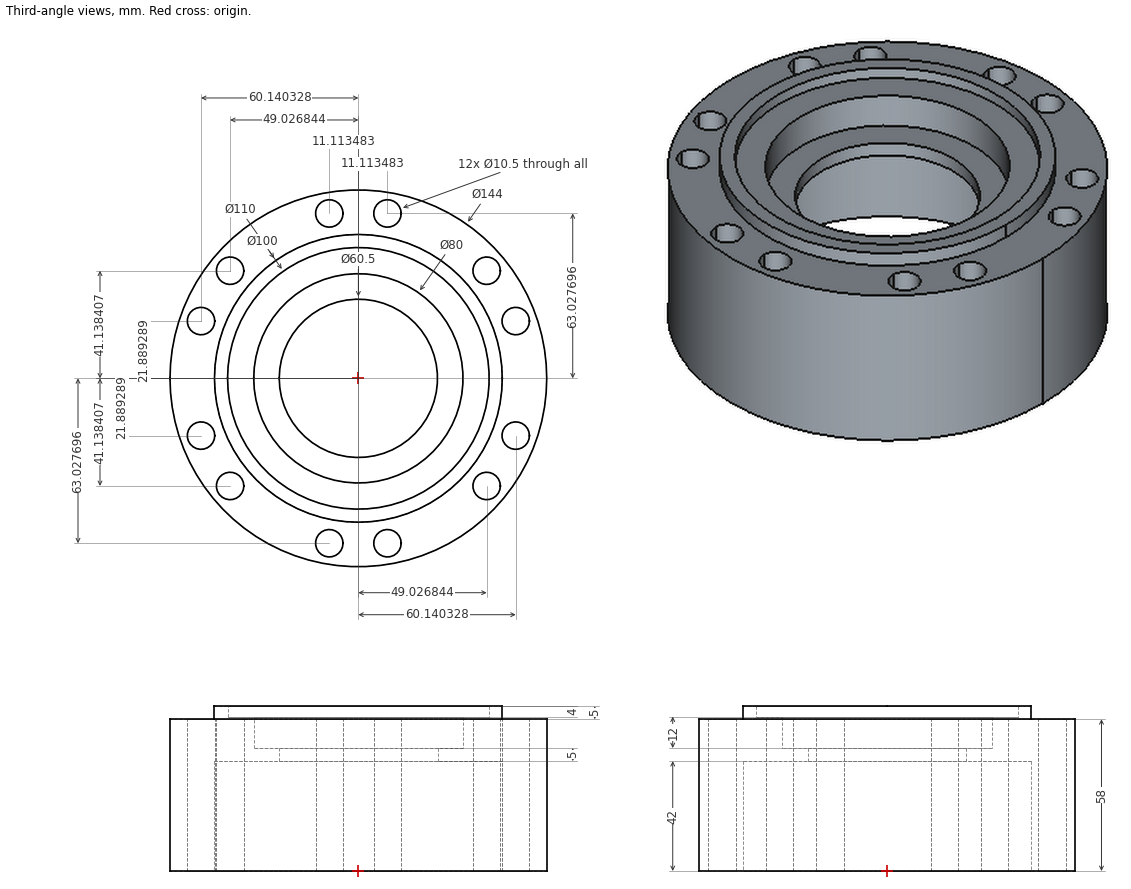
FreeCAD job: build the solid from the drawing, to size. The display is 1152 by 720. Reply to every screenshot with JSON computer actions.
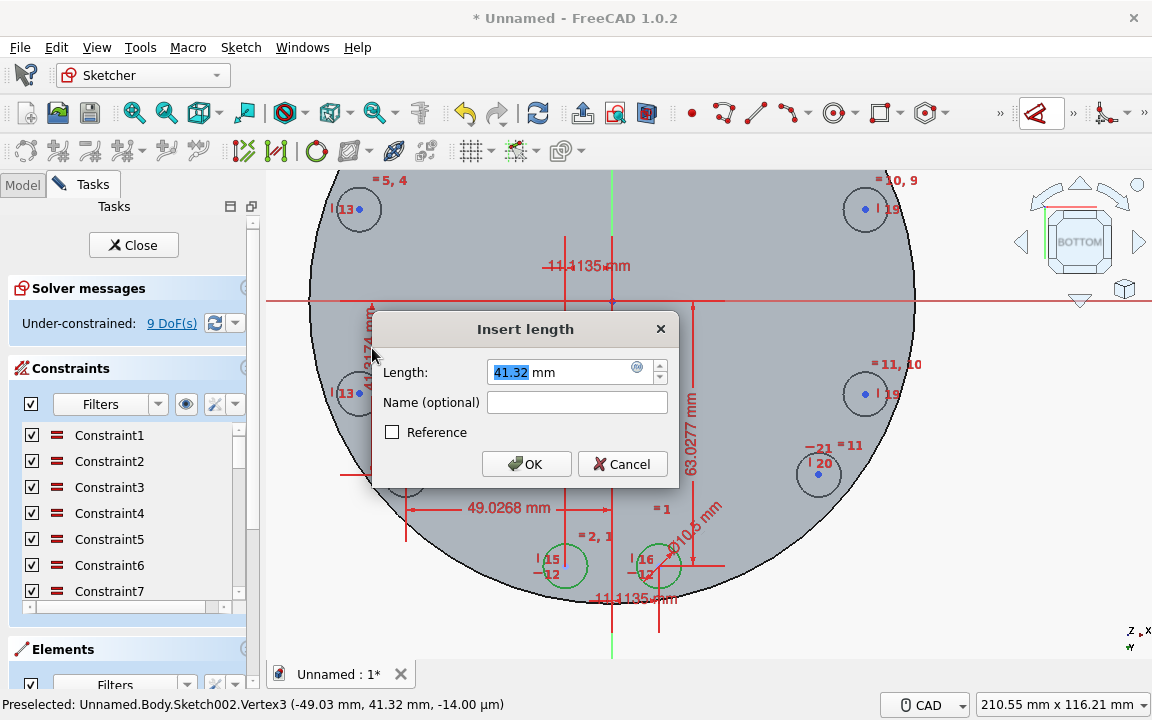
{"action": "type", "text": "41.138407"}
{"action": "key", "text": "Return"}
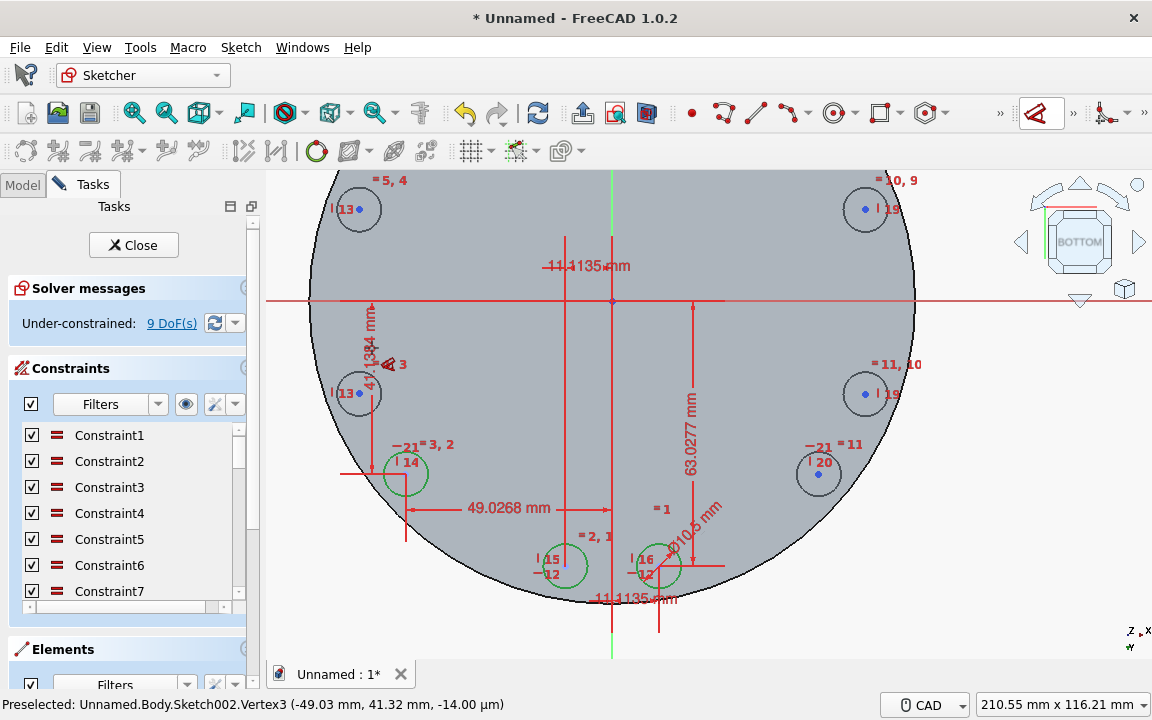
{"action": "left_click", "coordinate": [359, 394]}
{"action": "left_click", "coordinate": [486, 428]}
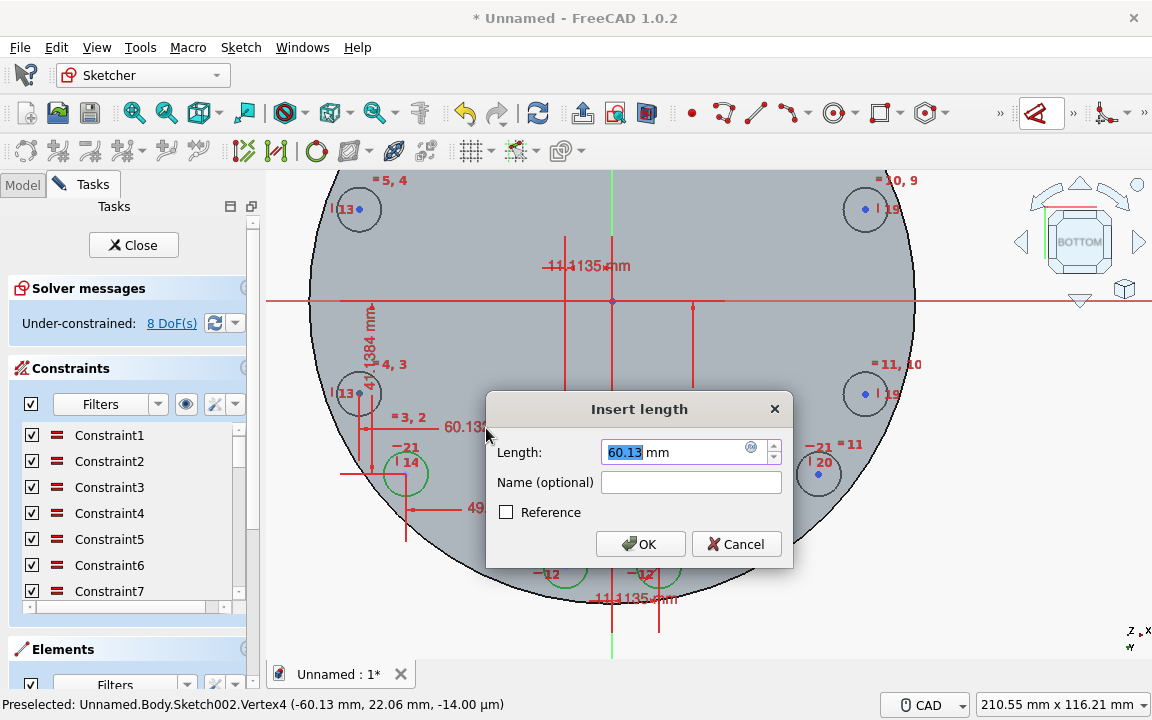
{"action": "type", "text": "60.140328"}
{"action": "key", "text": "Return"}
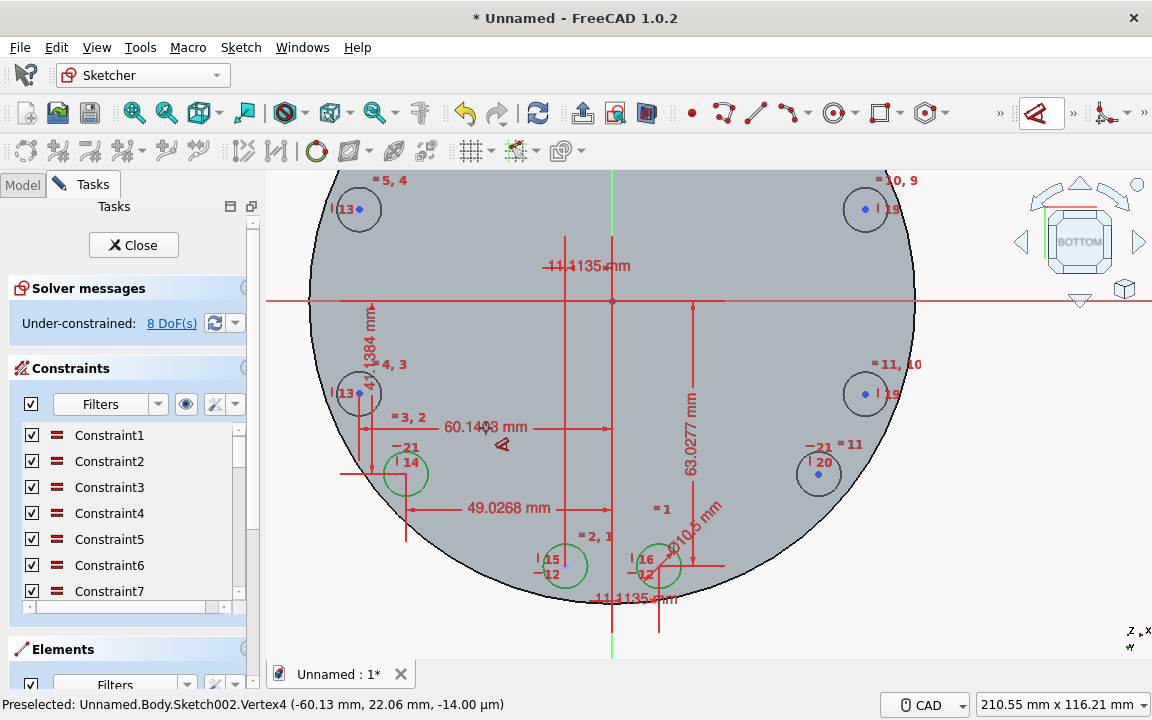
{"action": "left_click", "coordinate": [359, 394]}
{"action": "left_click", "coordinate": [325, 326]}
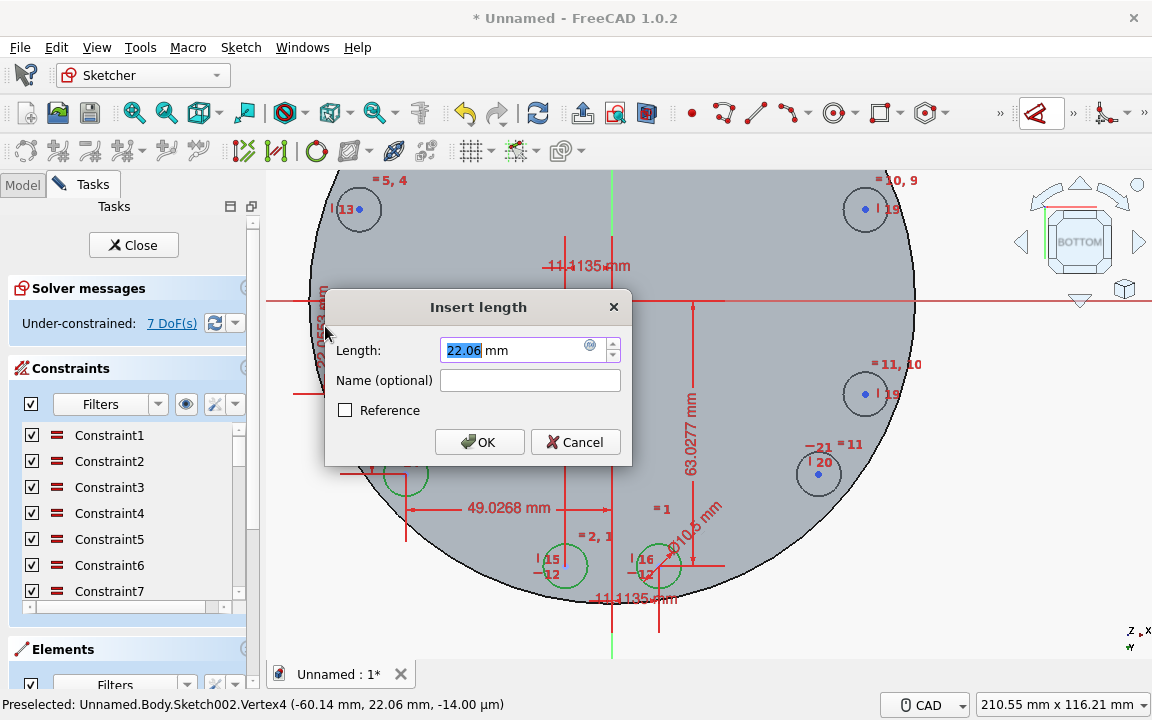
{"action": "type", "text": "21.889289"}
{"action": "key", "text": "Return"}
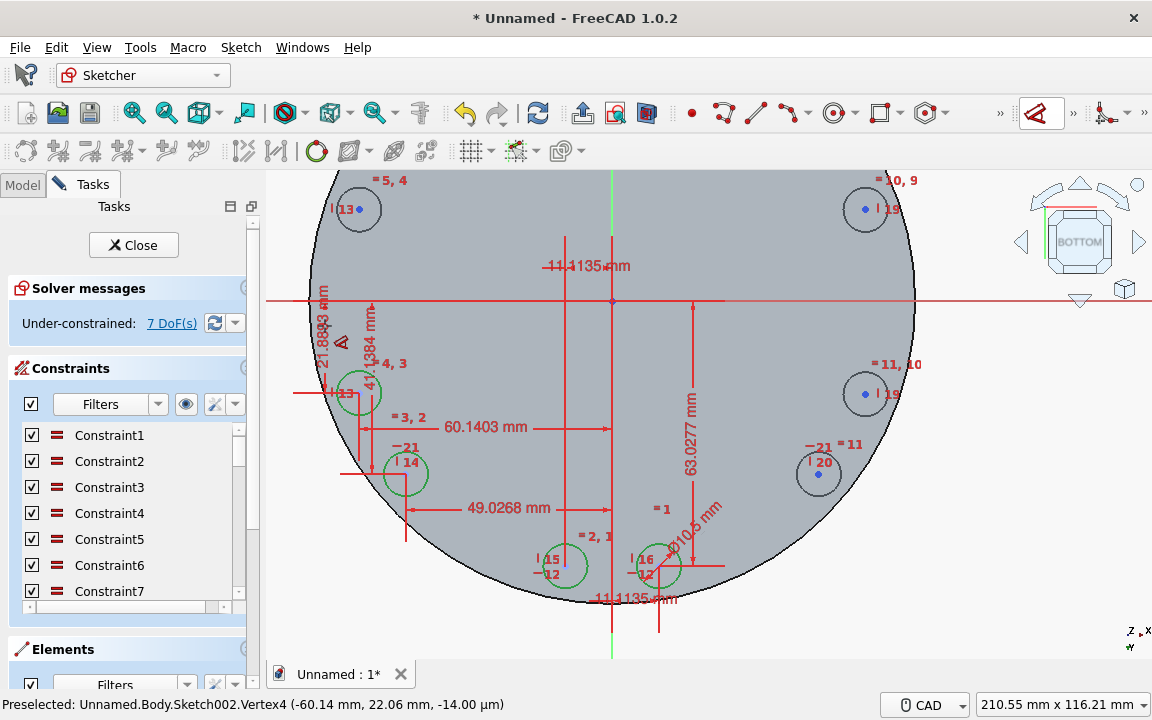
{"action": "left_click", "coordinate": [359, 210]}
{"action": "left_click", "coordinate": [325, 255]}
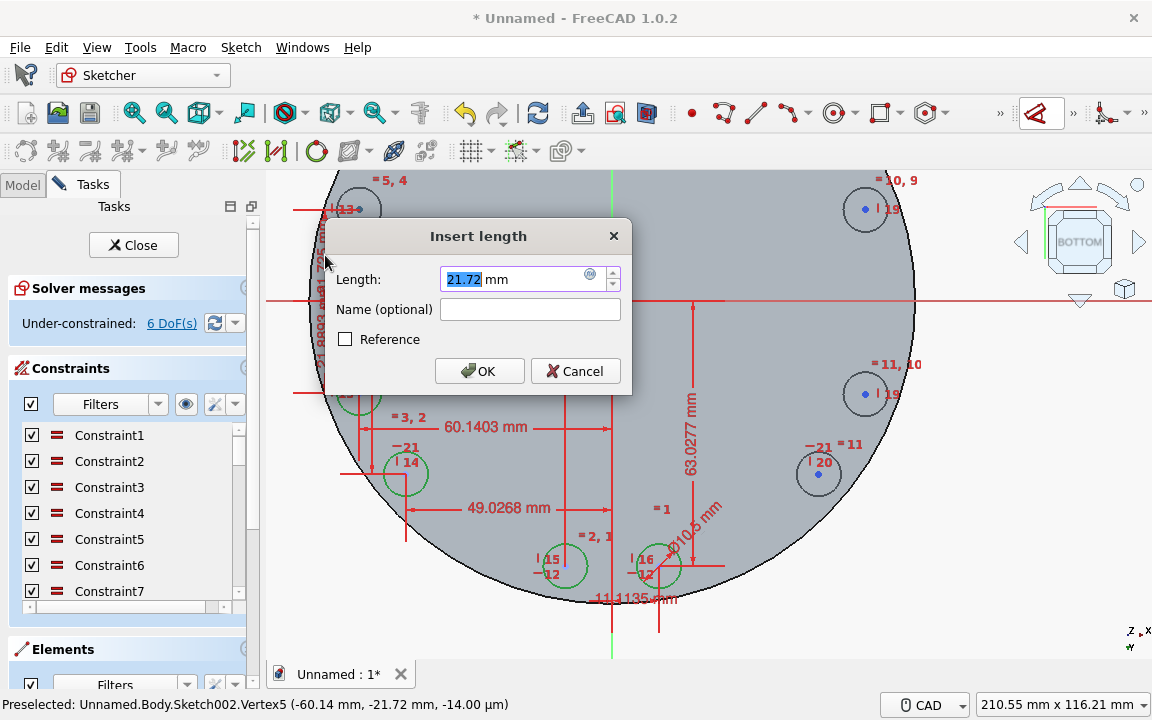
{"action": "type", "text": "21.889289"}
{"action": "key", "text": "Return"}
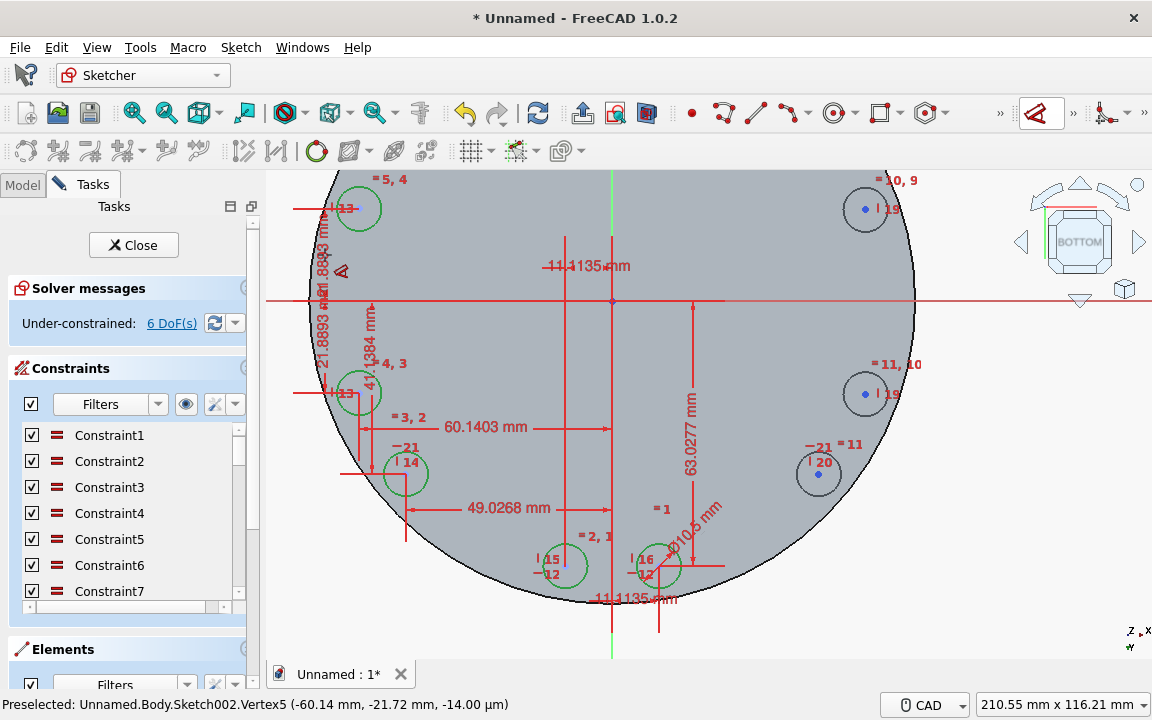
{"action": "scroll", "coordinate": [675, 553], "scroll_direction": "down", "scroll_amount": 3}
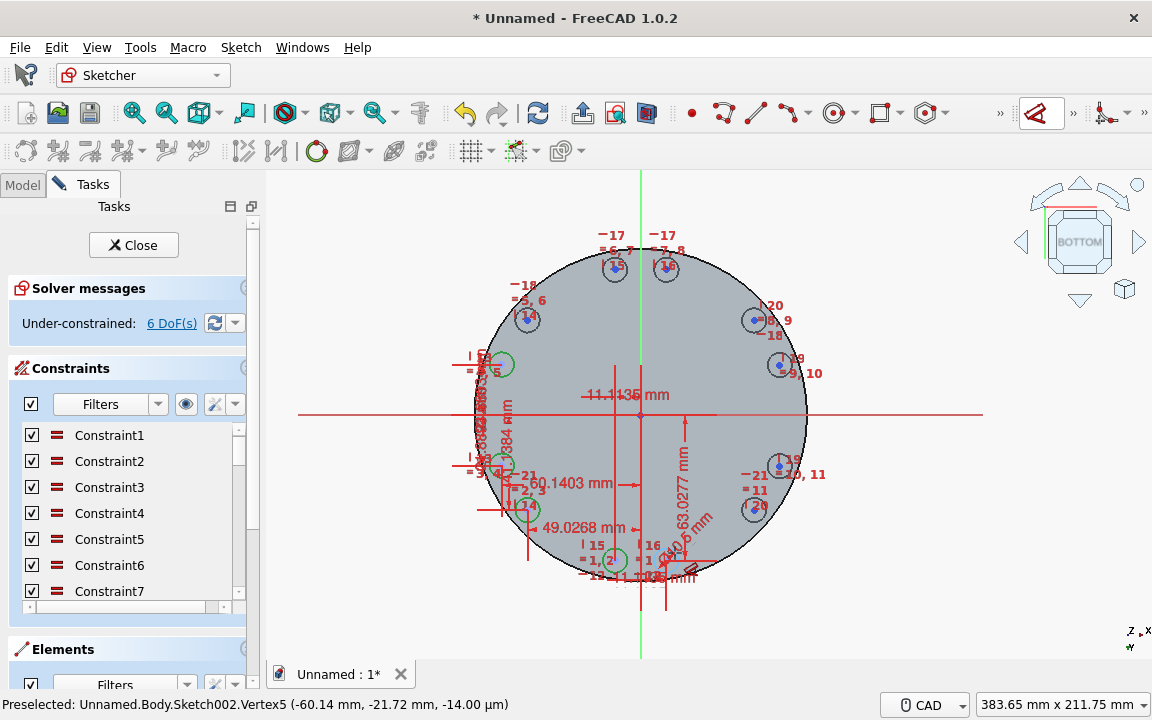
{"action": "left_click", "coordinate": [528, 320]}
{"action": "left_click", "coordinate": [494, 335]}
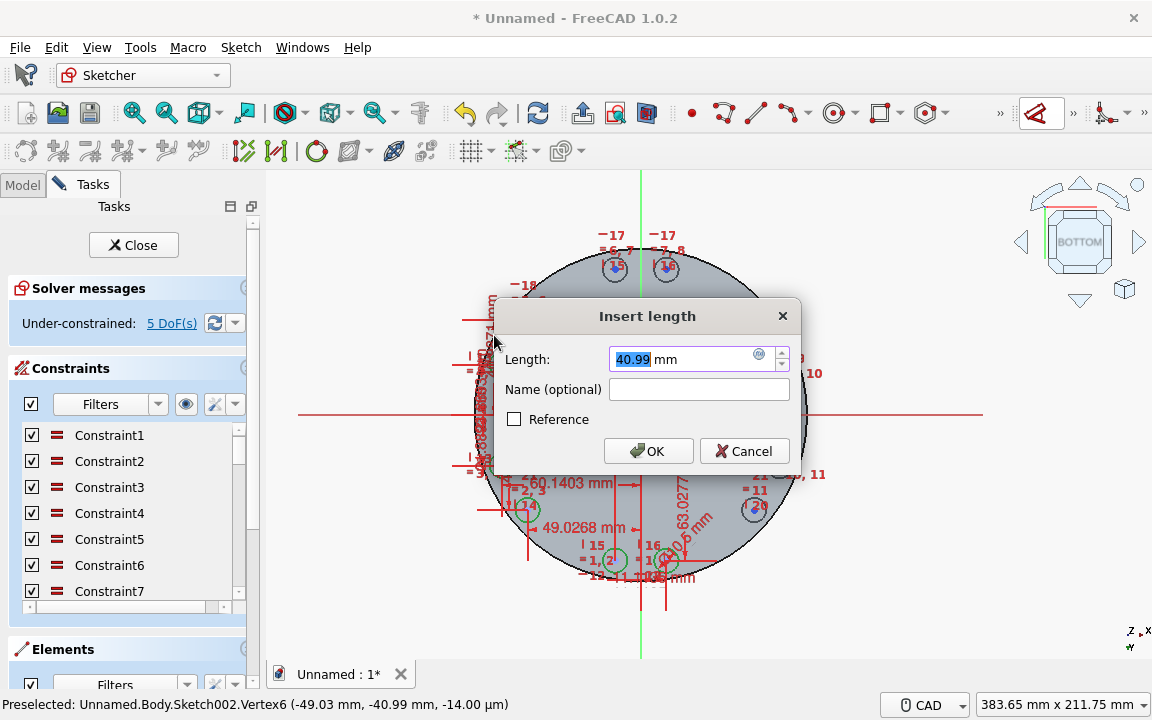
{"action": "type", "text": "41.138407"}
{"action": "key", "text": "Return"}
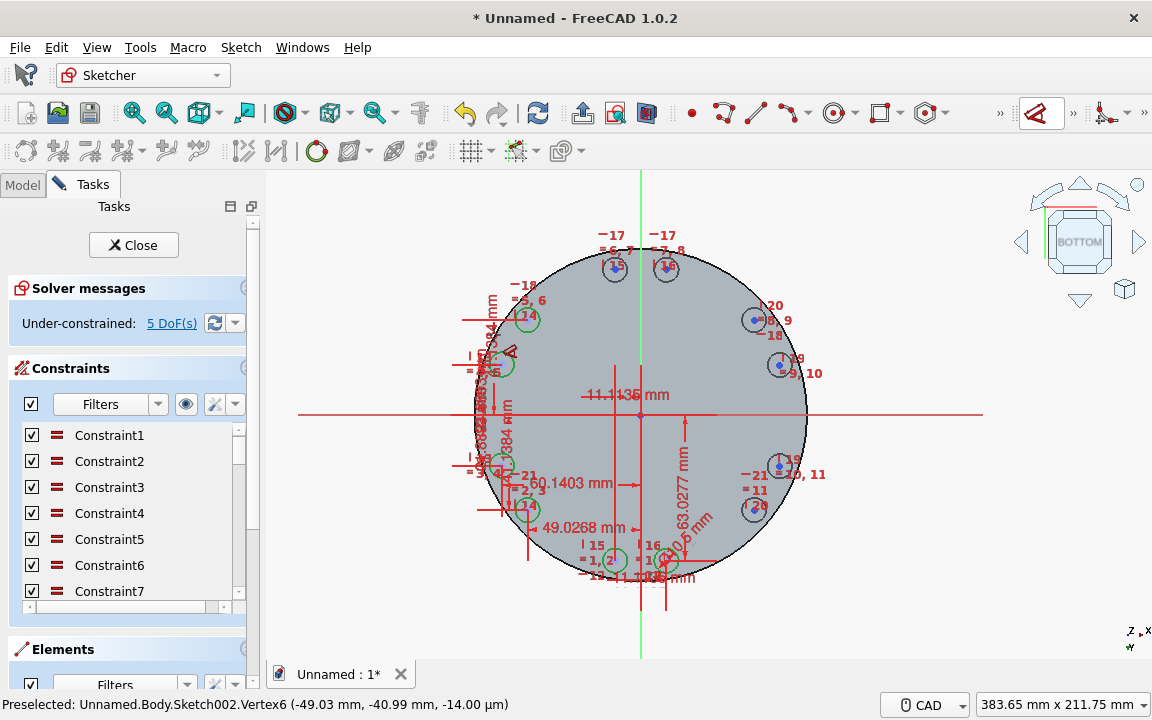
{"action": "left_click", "coordinate": [615, 270]}
{"action": "left_click", "coordinate": [581, 342]}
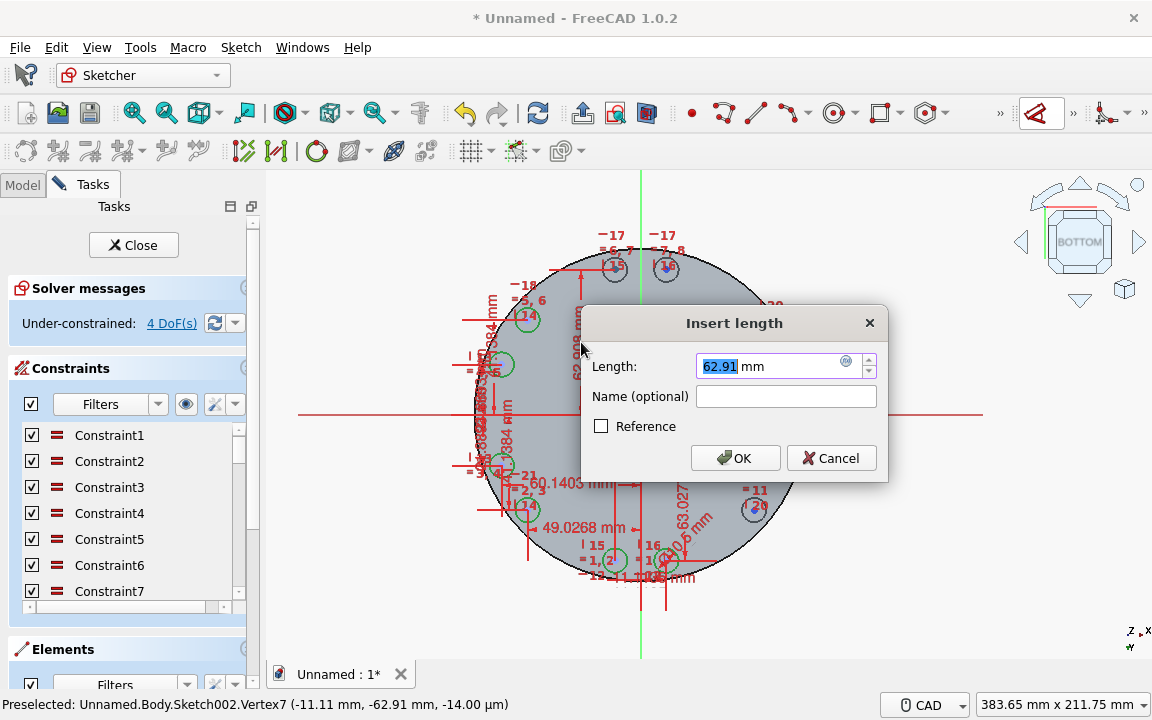
{"action": "type", "text": "63.027696"}
{"action": "key", "text": "Return"}